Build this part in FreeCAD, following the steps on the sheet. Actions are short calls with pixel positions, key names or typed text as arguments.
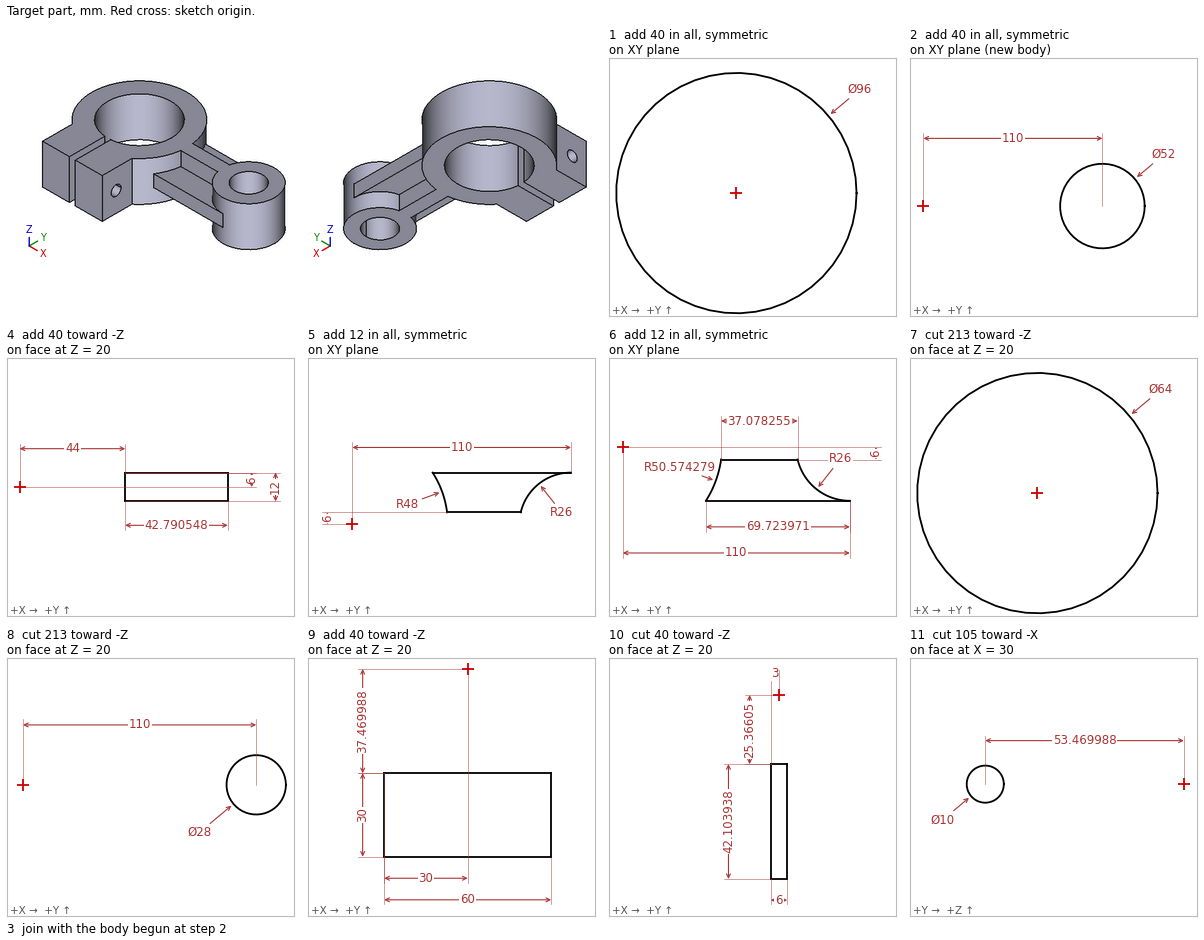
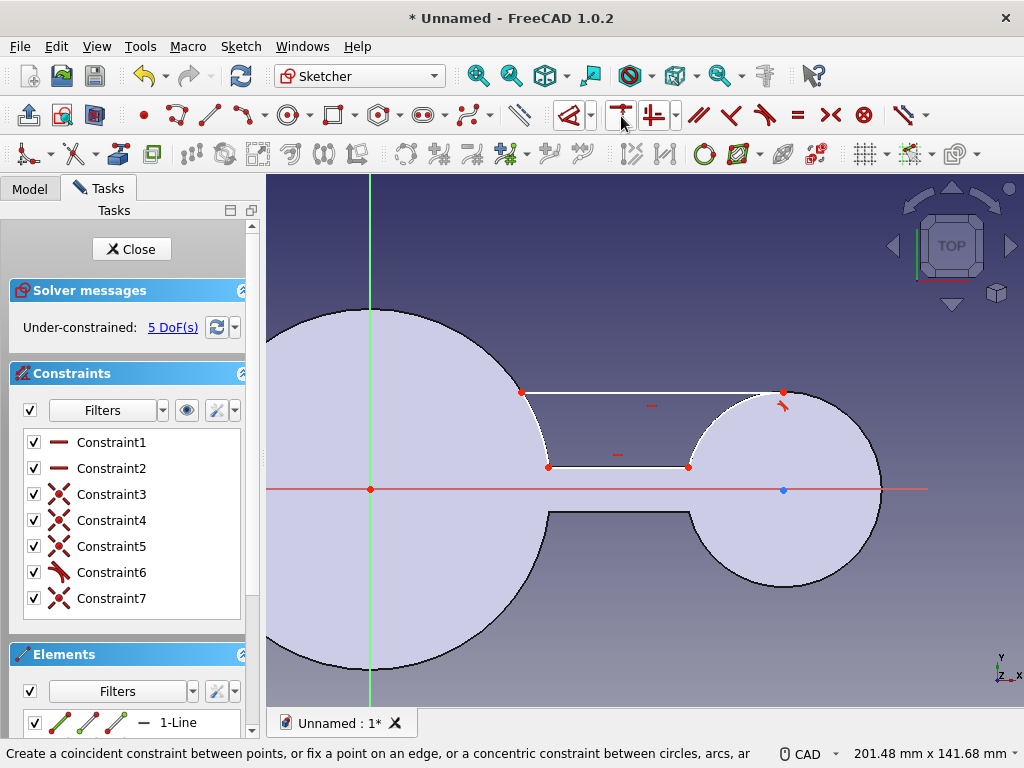
click(784, 490)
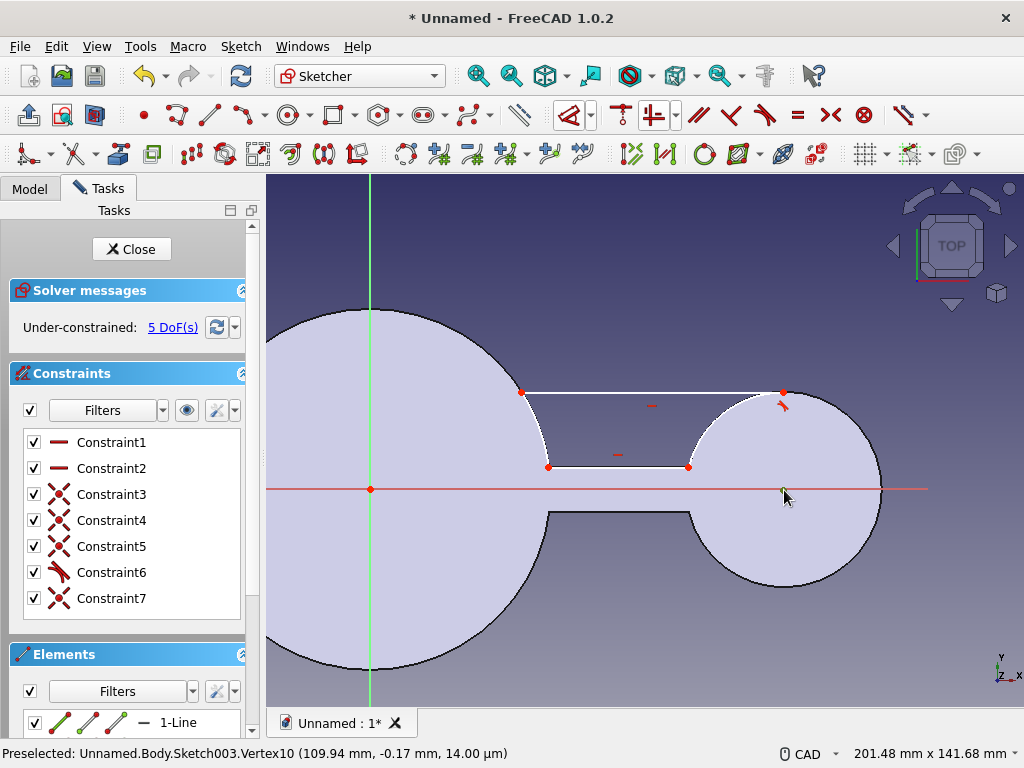
click(334, 489)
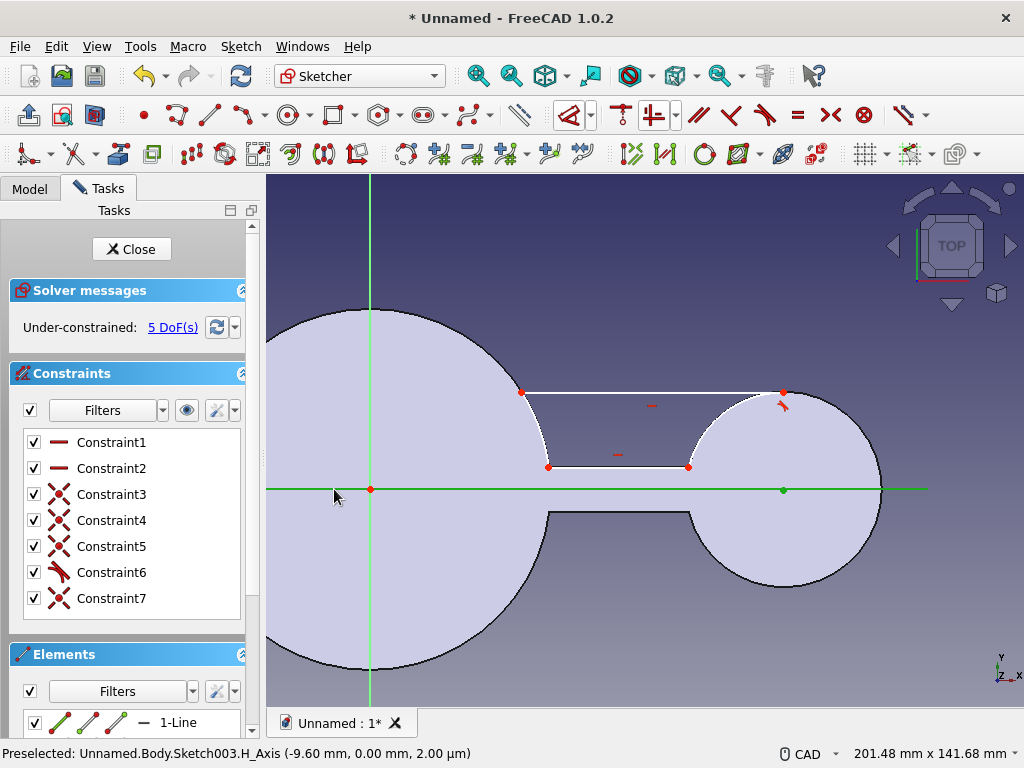
click(621, 116)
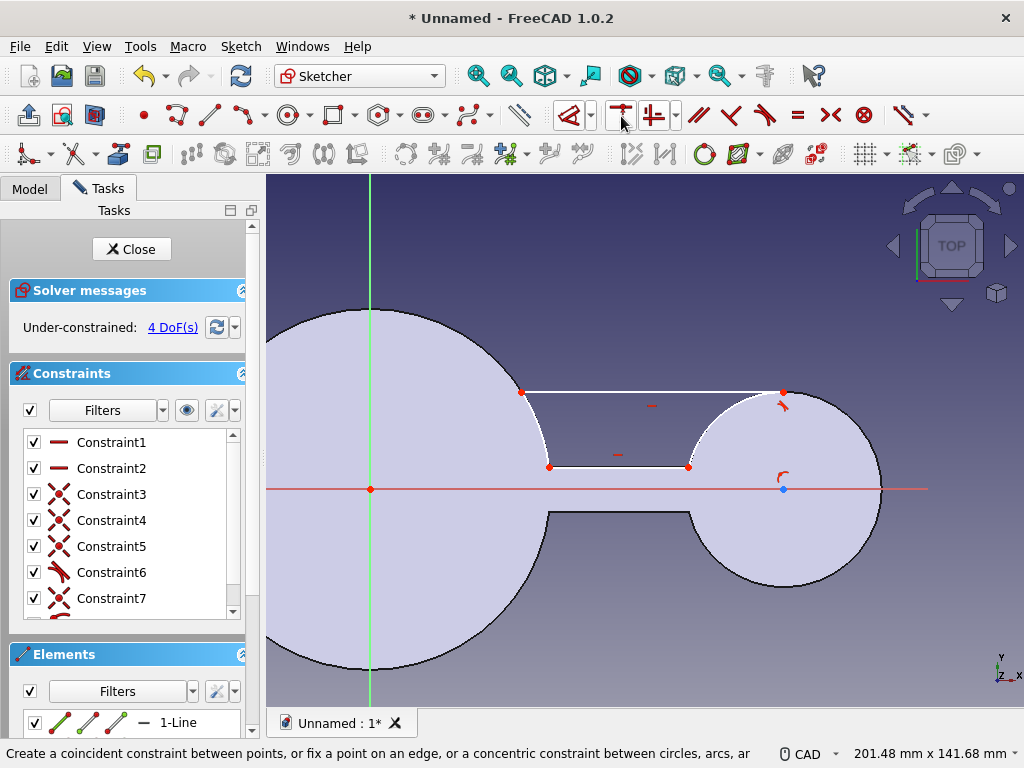
click(545, 444)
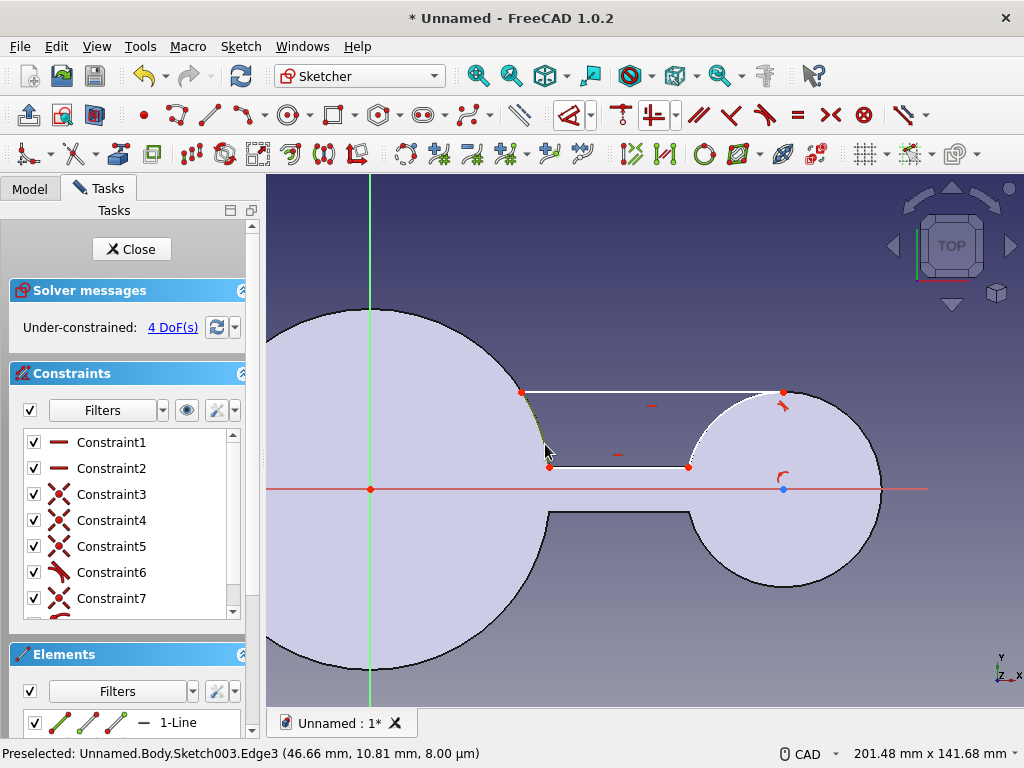
key(k)
key(r)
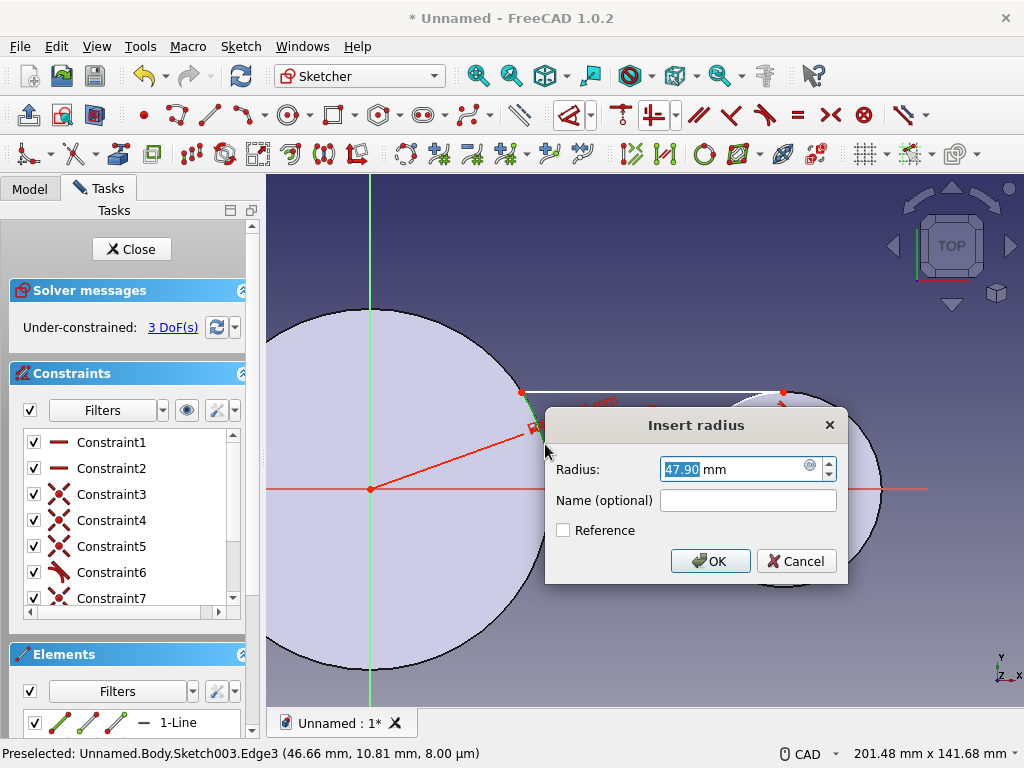
text(48)
key(Return)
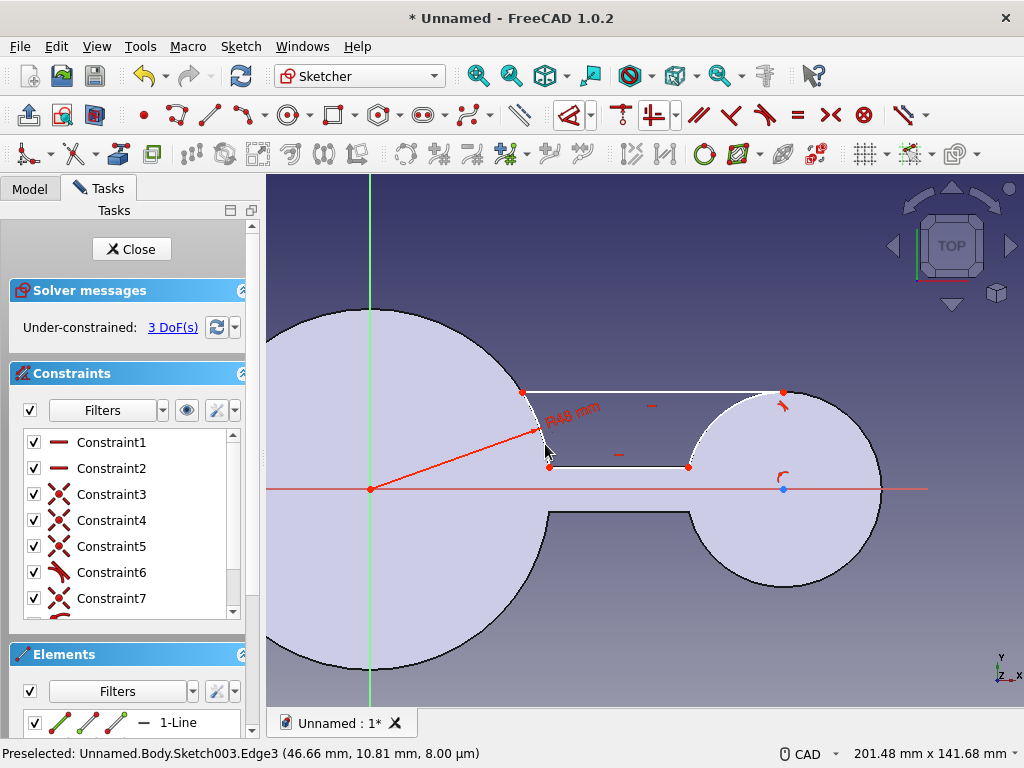
click(705, 432)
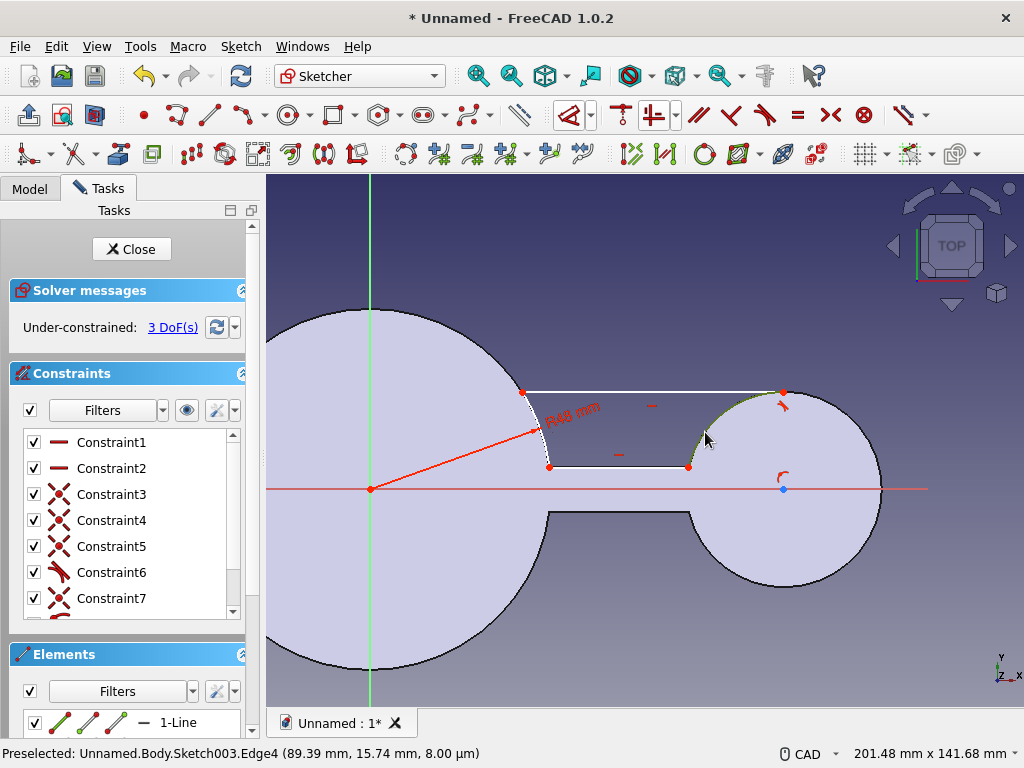
key(k)
key(r)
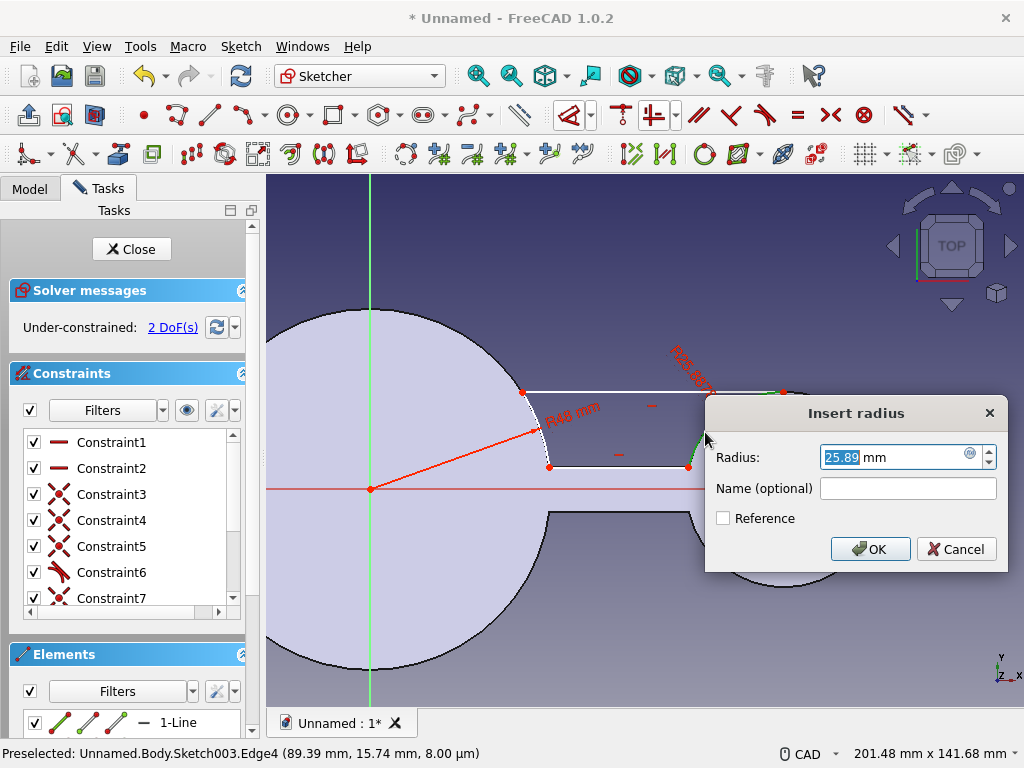
text(26)
key(Return)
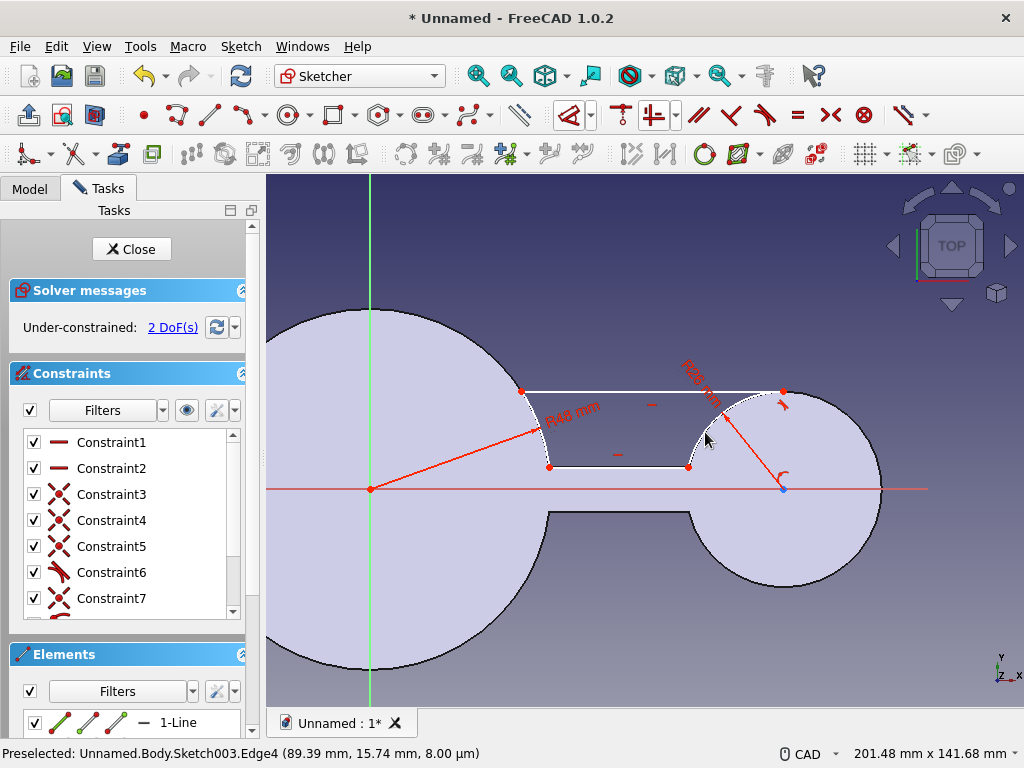
scroll(549, 468, up, 3)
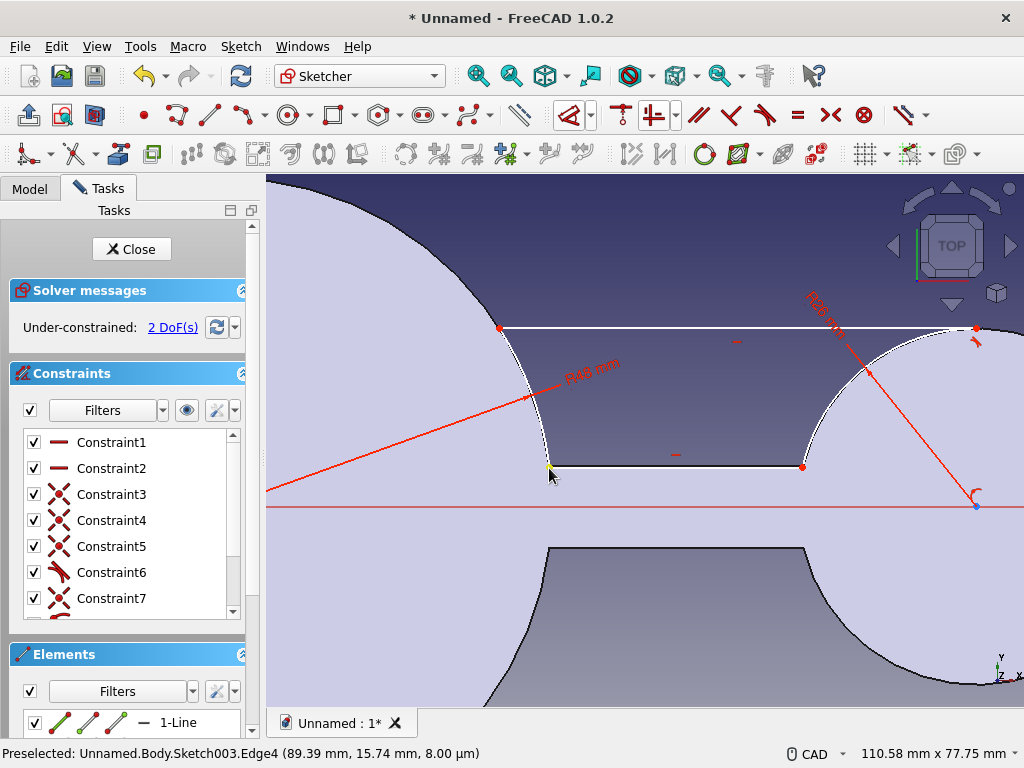
click(549, 468)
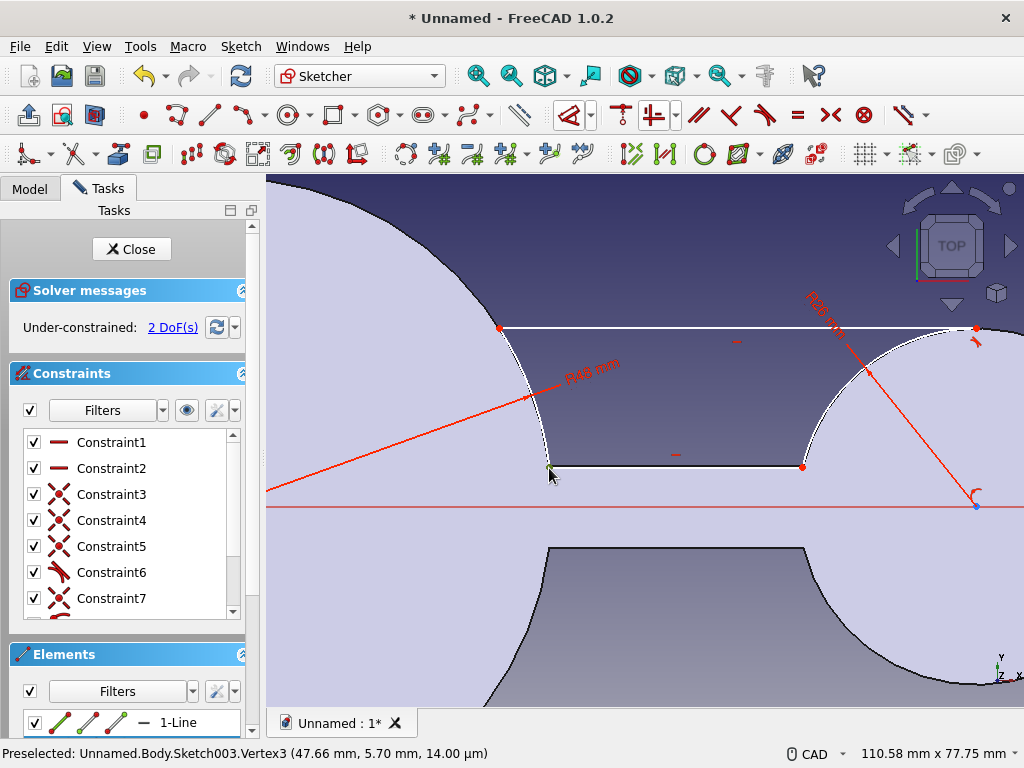
click(590, 116)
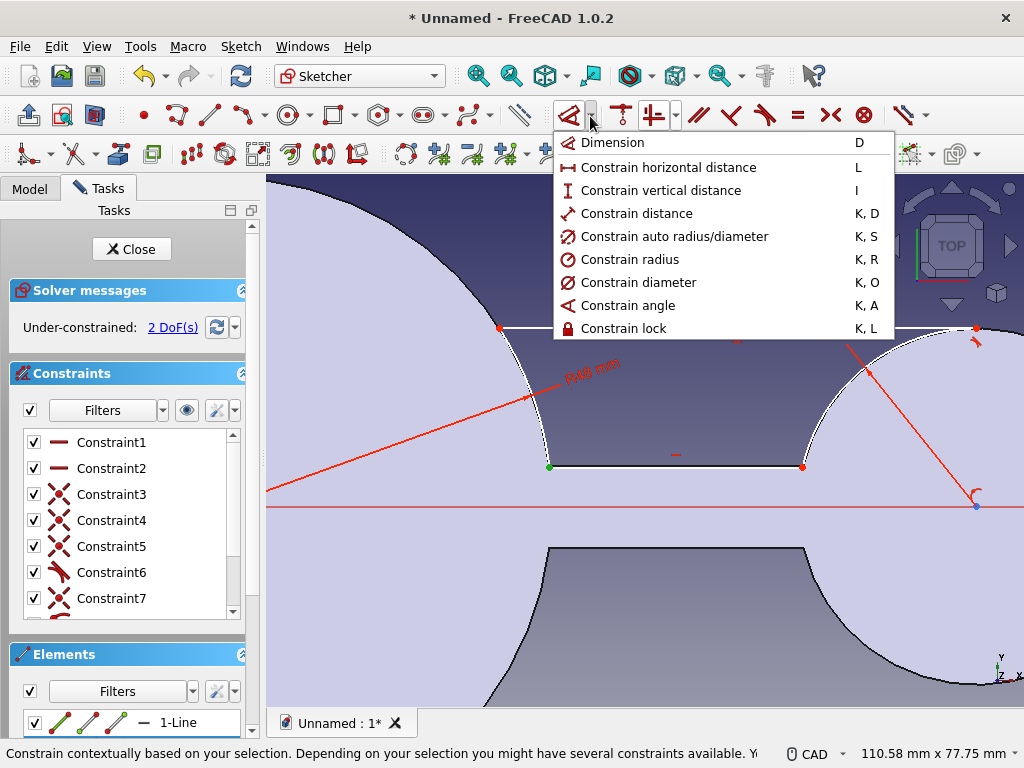
click(724, 190)